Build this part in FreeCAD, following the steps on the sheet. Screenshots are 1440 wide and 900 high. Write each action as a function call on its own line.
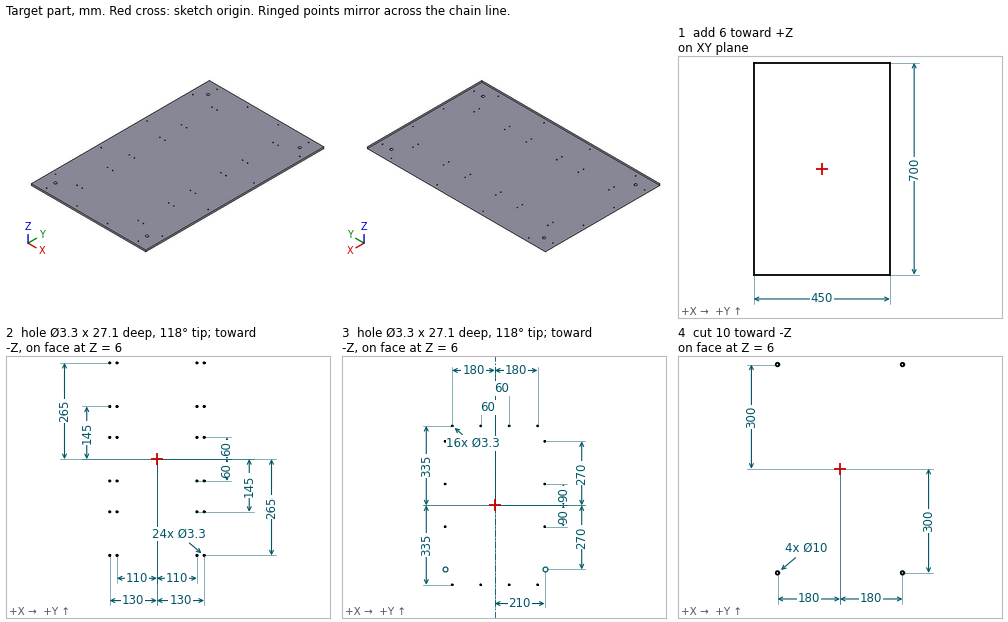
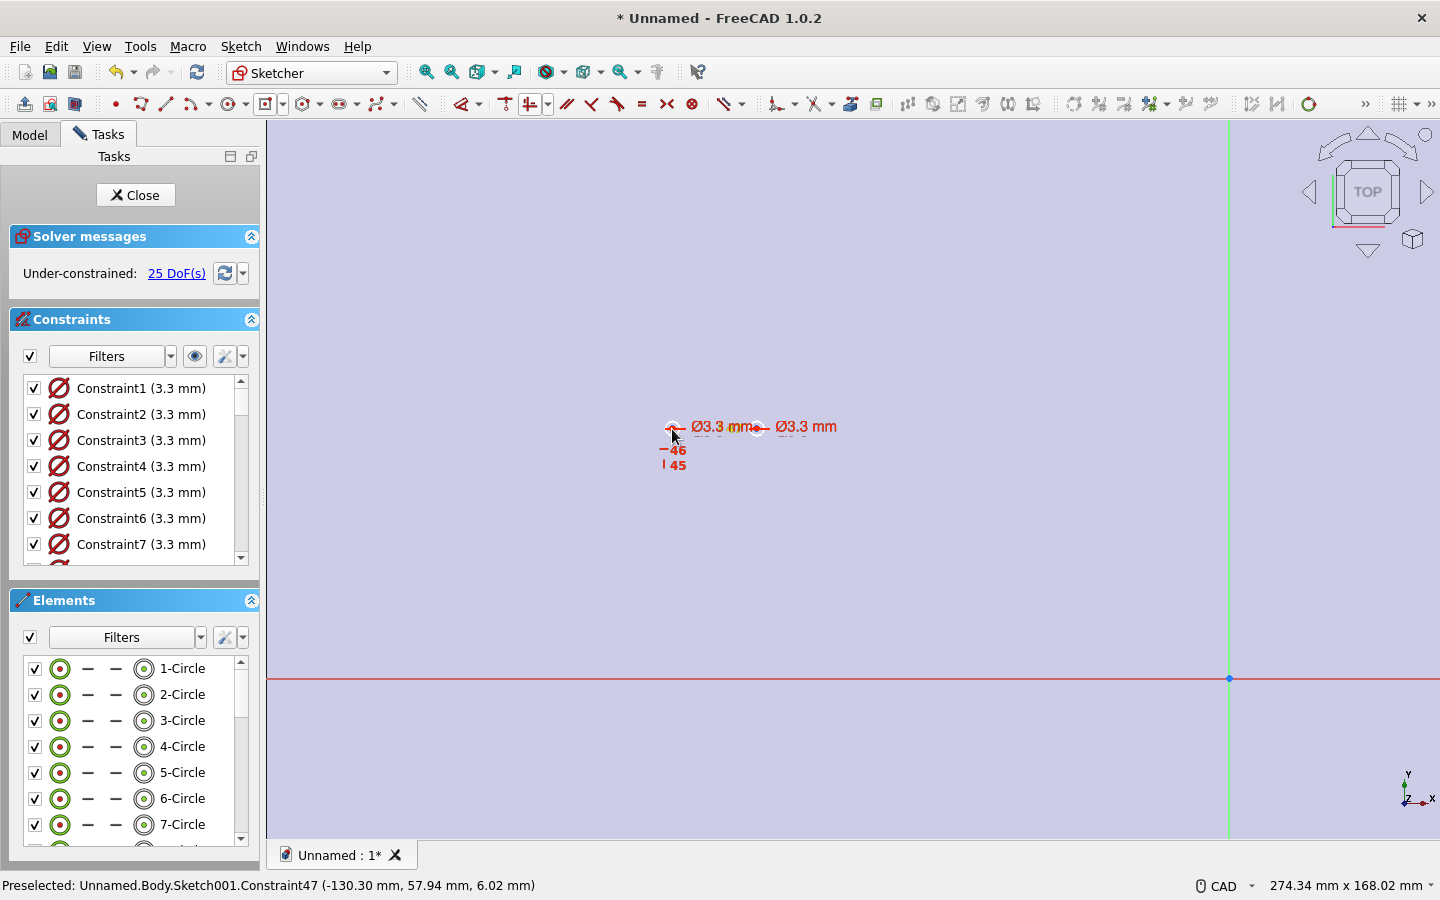
click(673, 429)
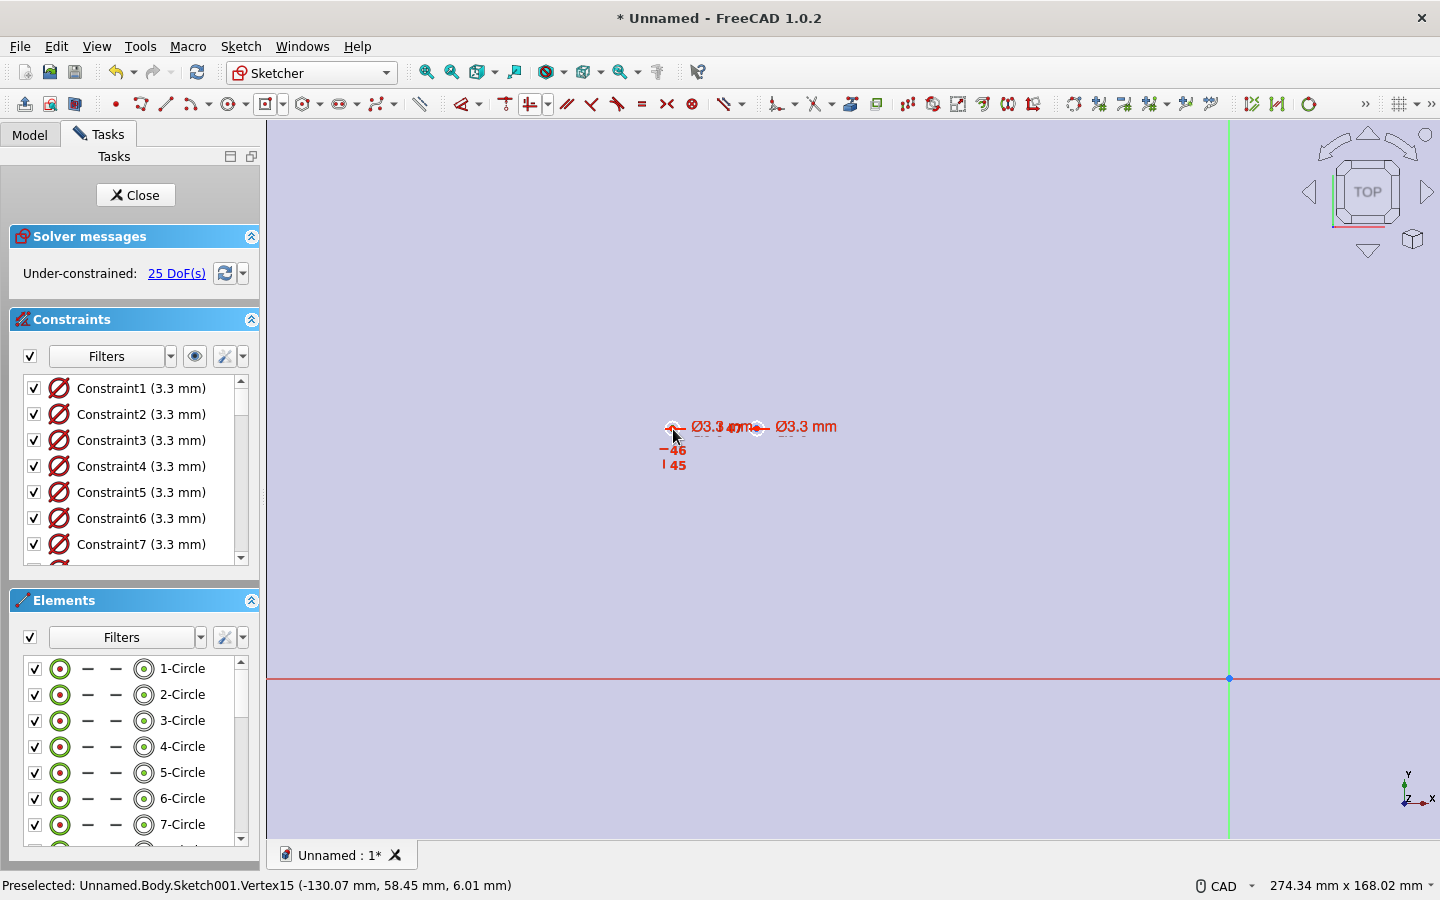
scroll(672, 429, down, 8)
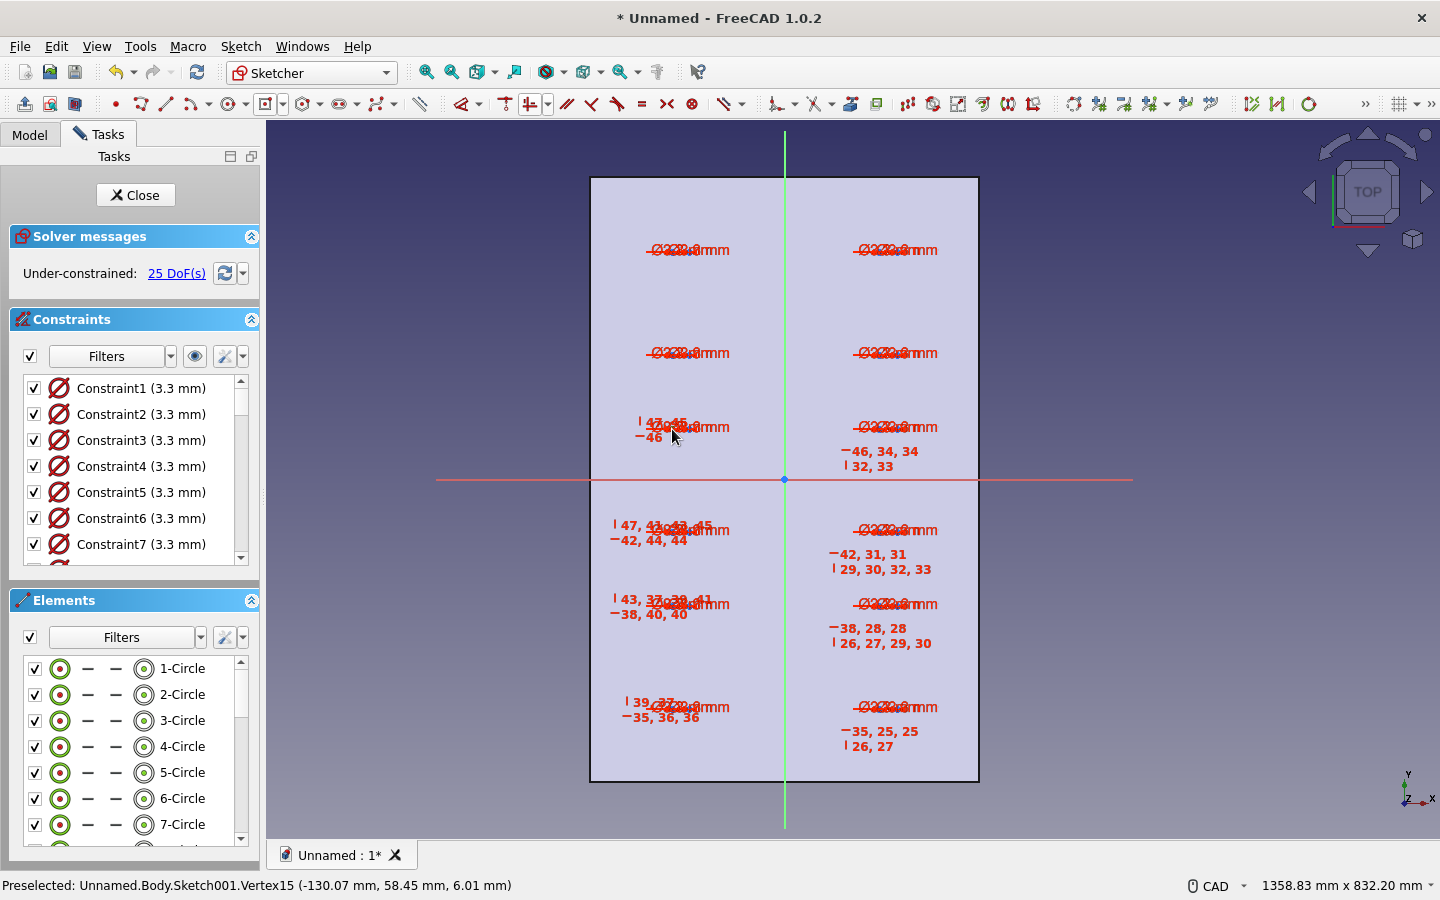
click(689, 429)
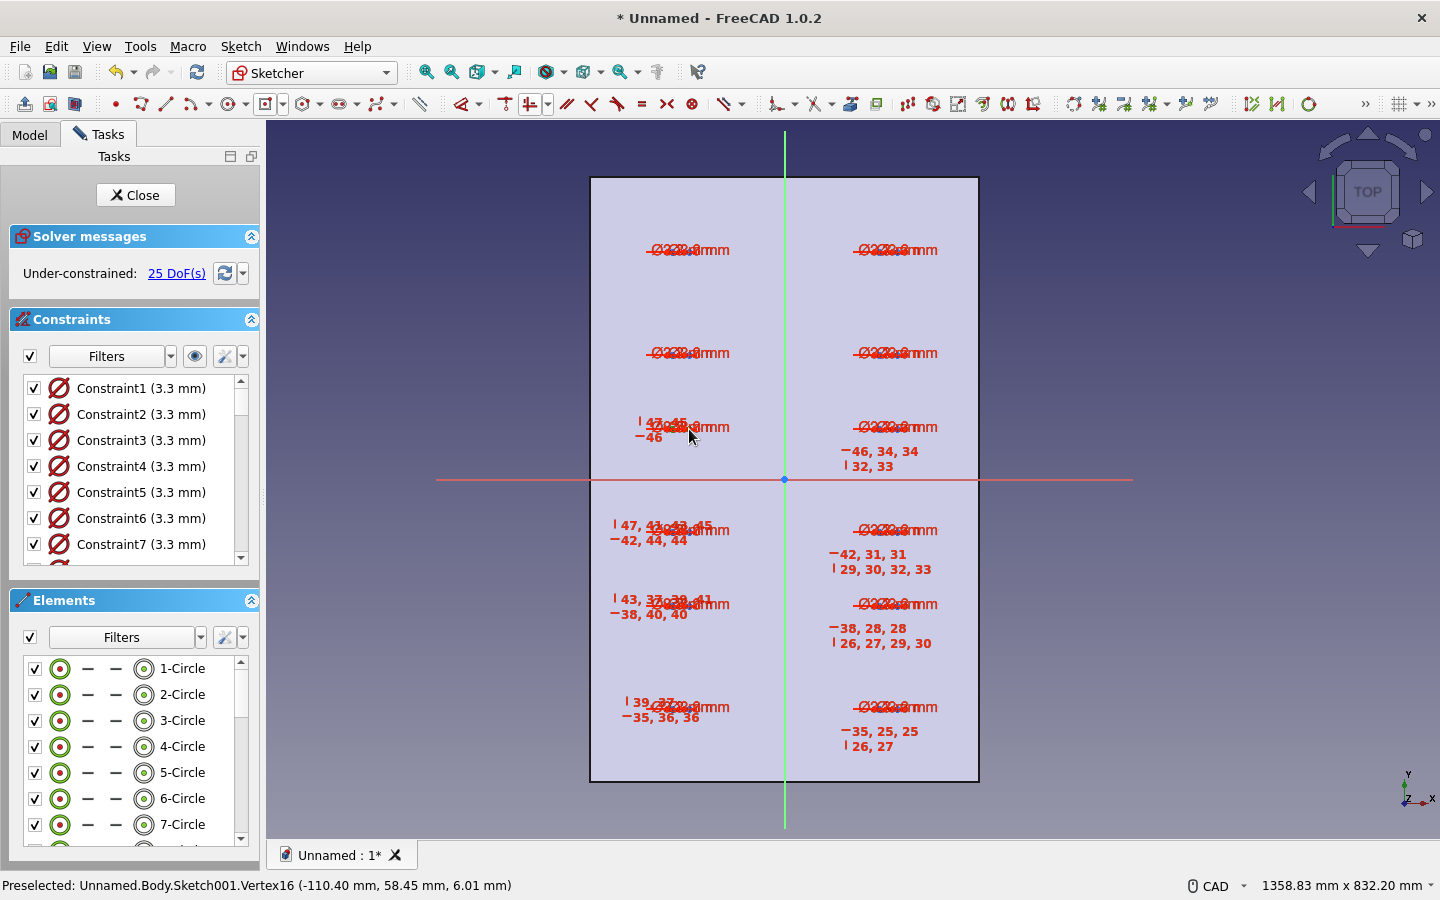
click(548, 104)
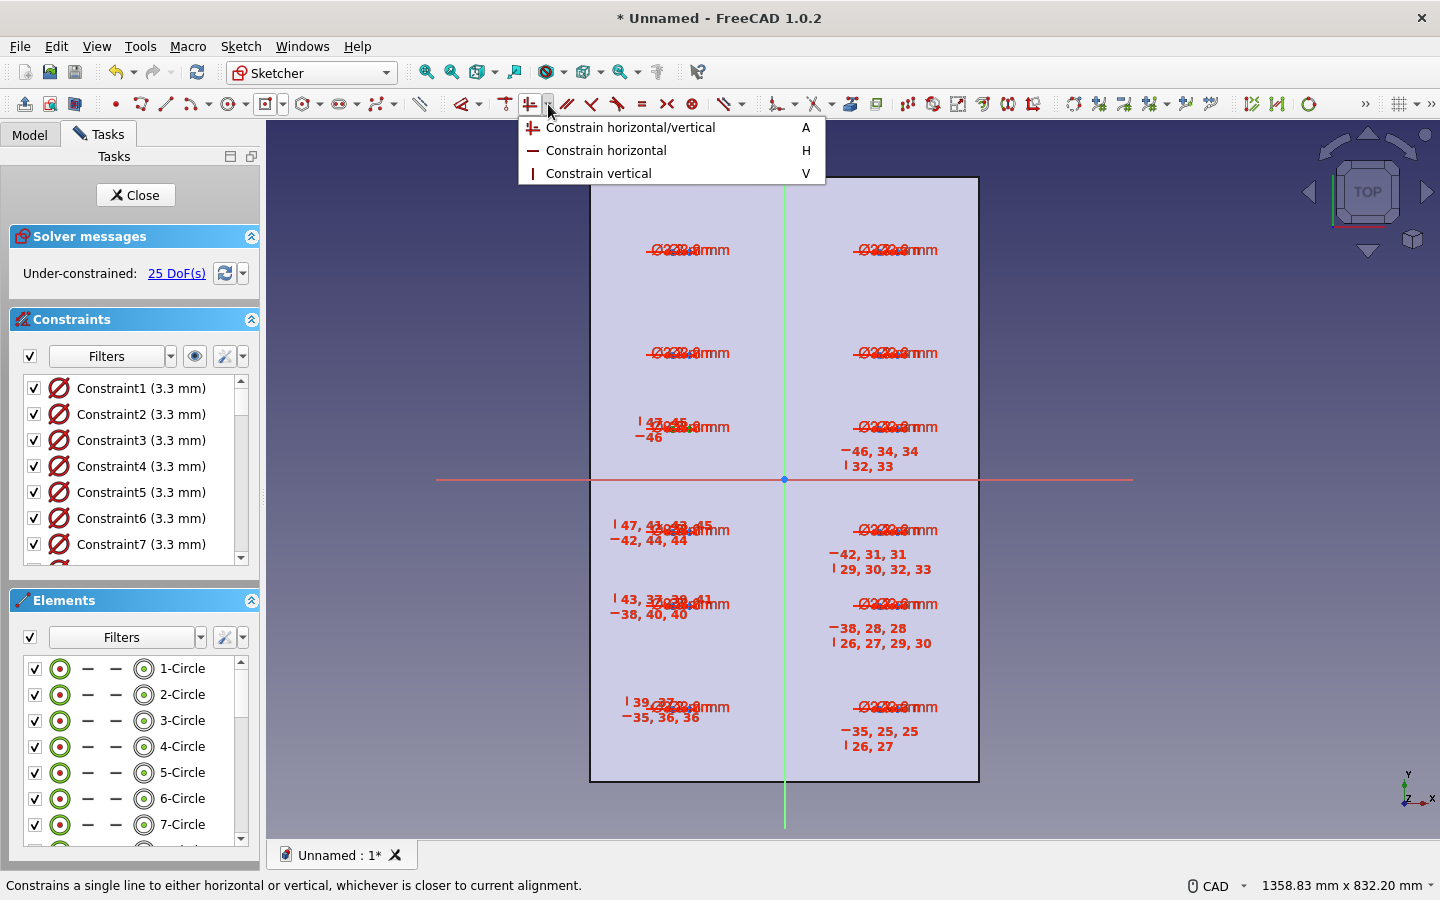
click(672, 150)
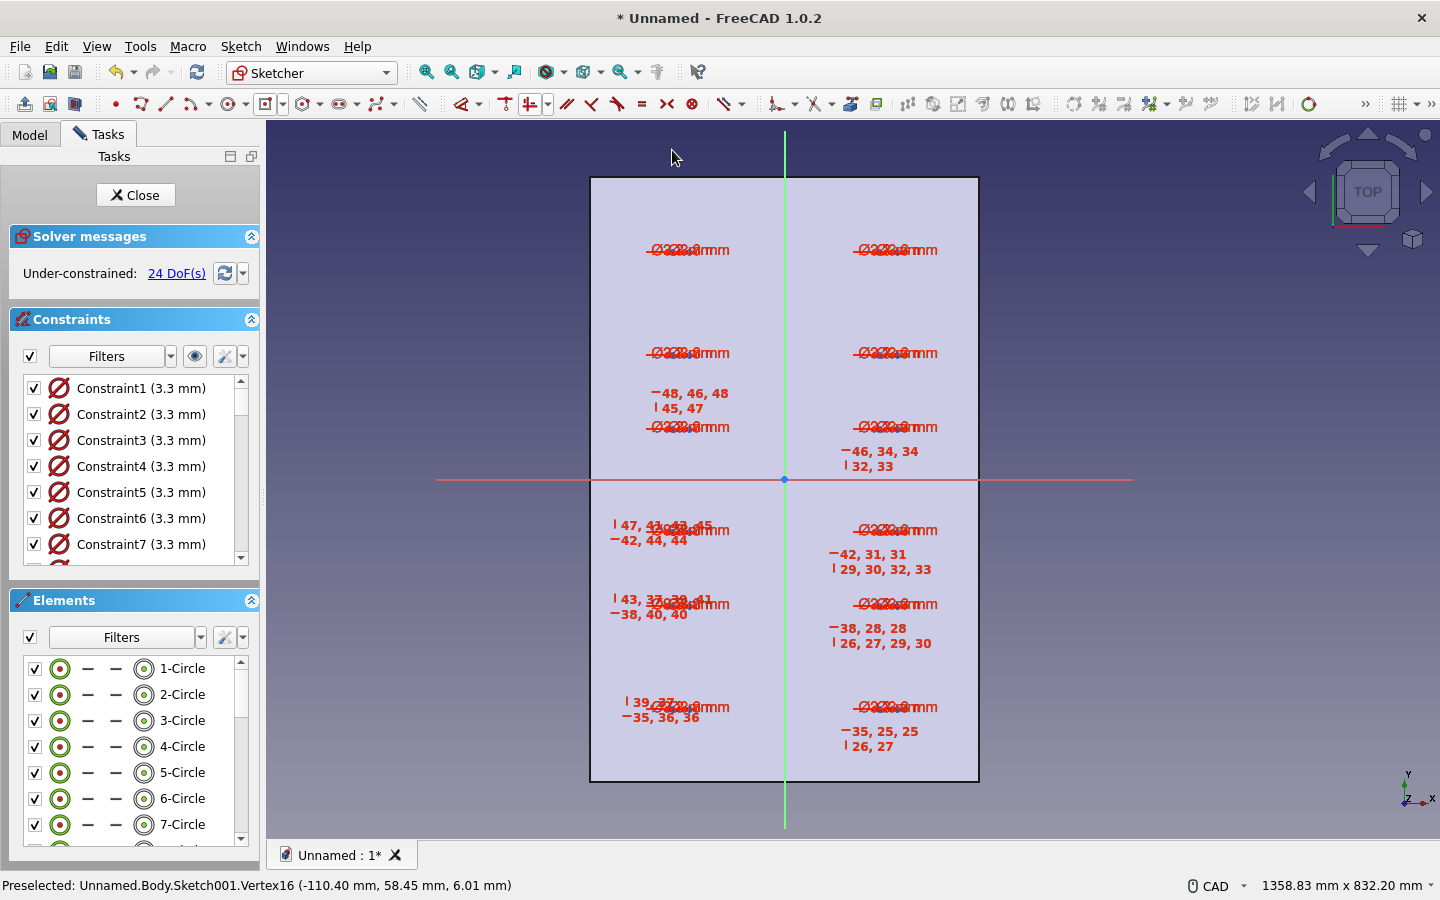
click(672, 429)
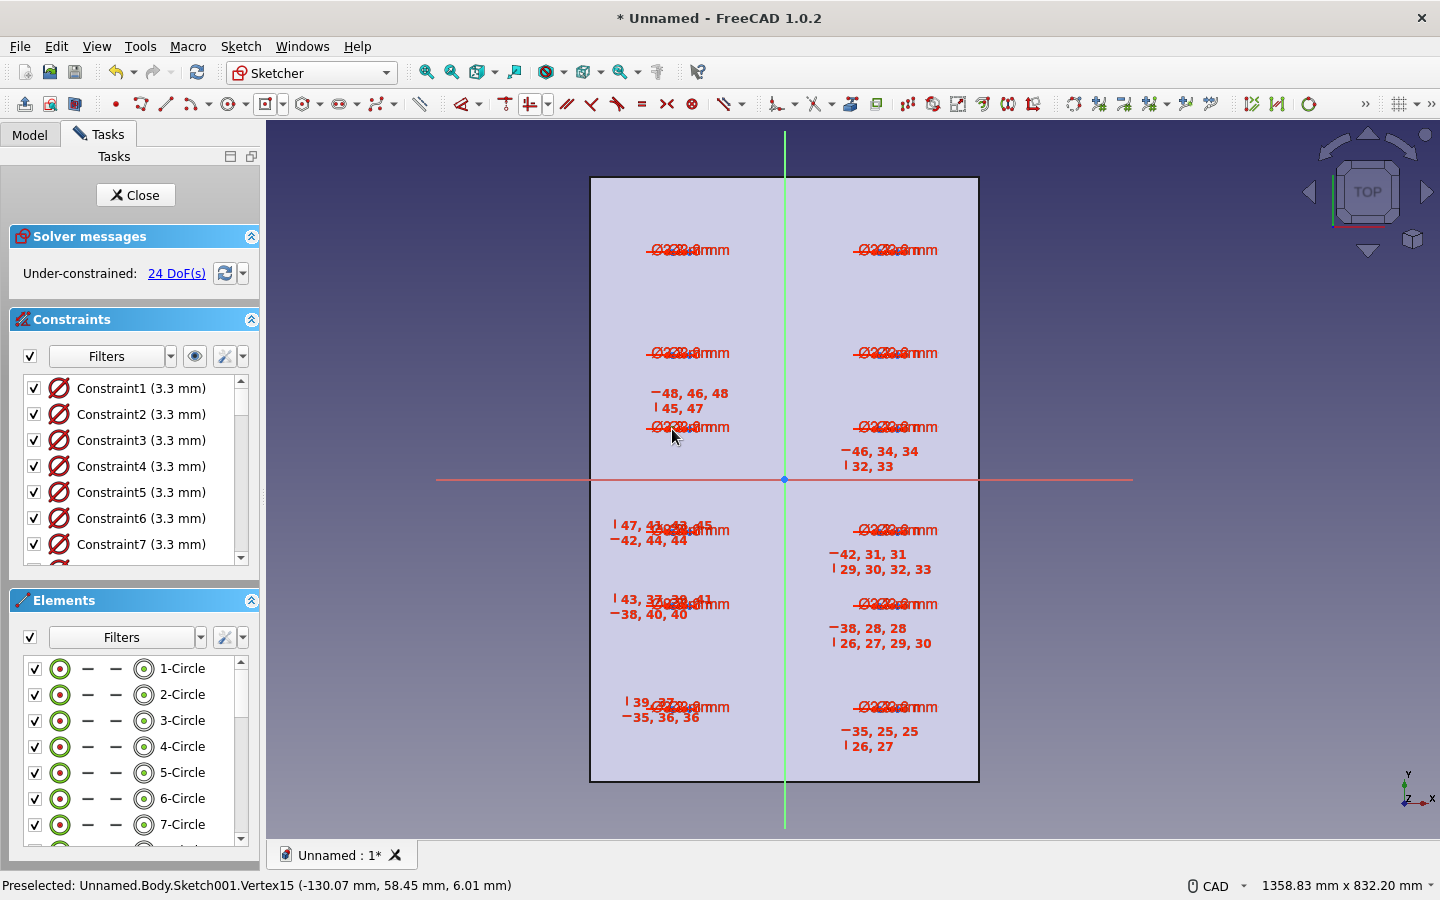
click(672, 355)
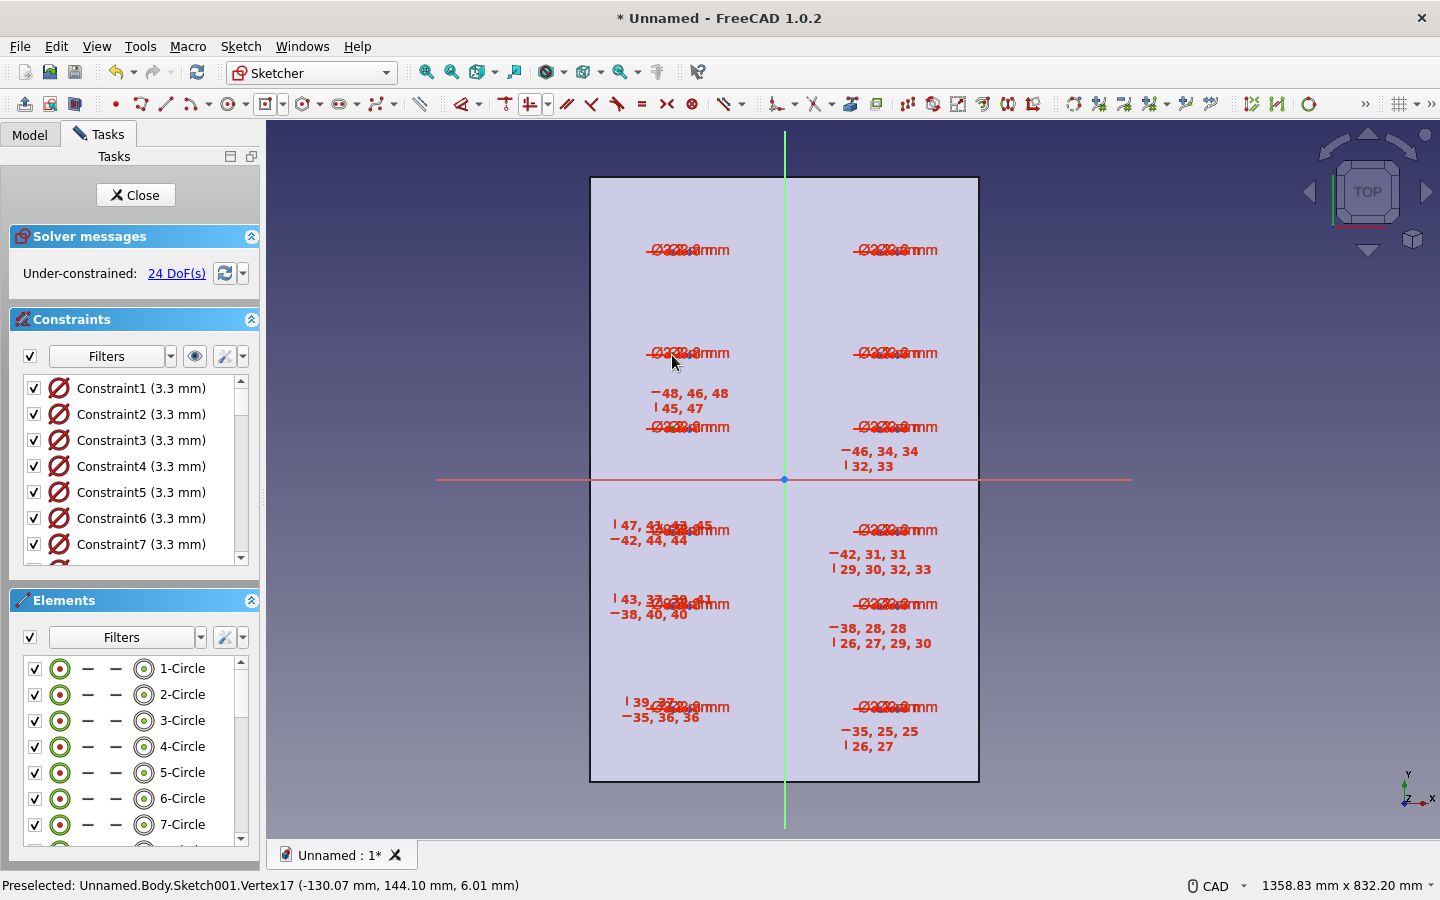
key(v)